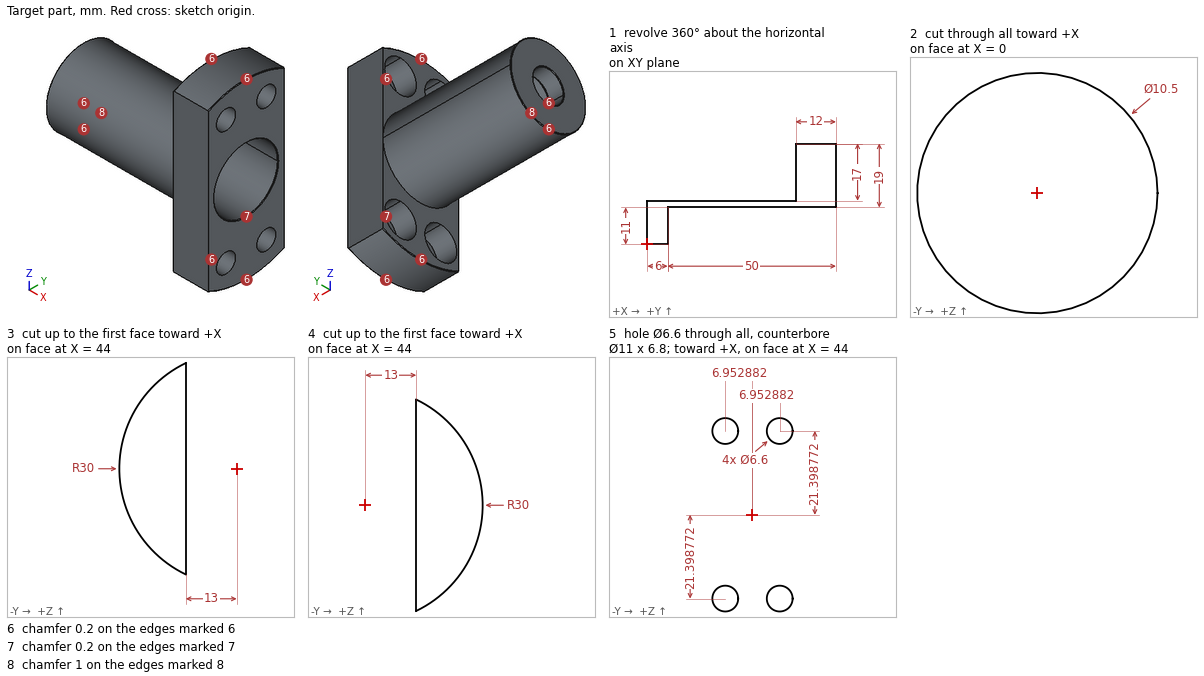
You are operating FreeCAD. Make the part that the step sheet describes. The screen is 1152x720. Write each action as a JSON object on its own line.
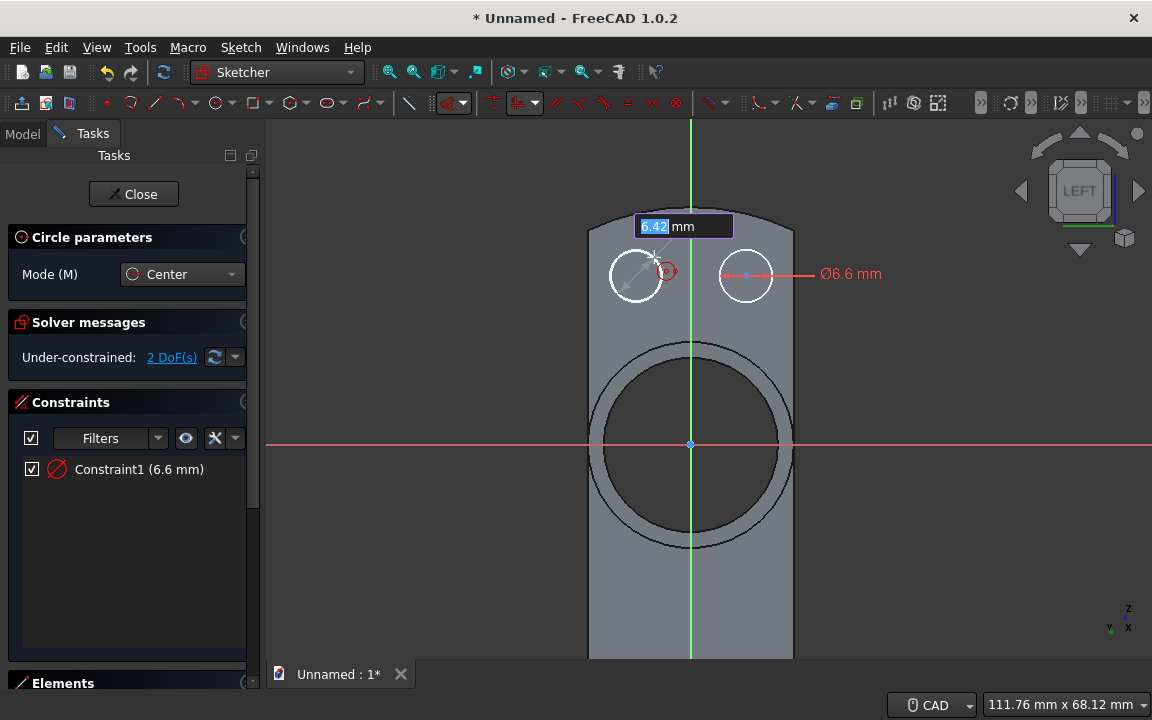
{"action": "type", "text": "6.6"}
{"action": "key", "text": "Return"}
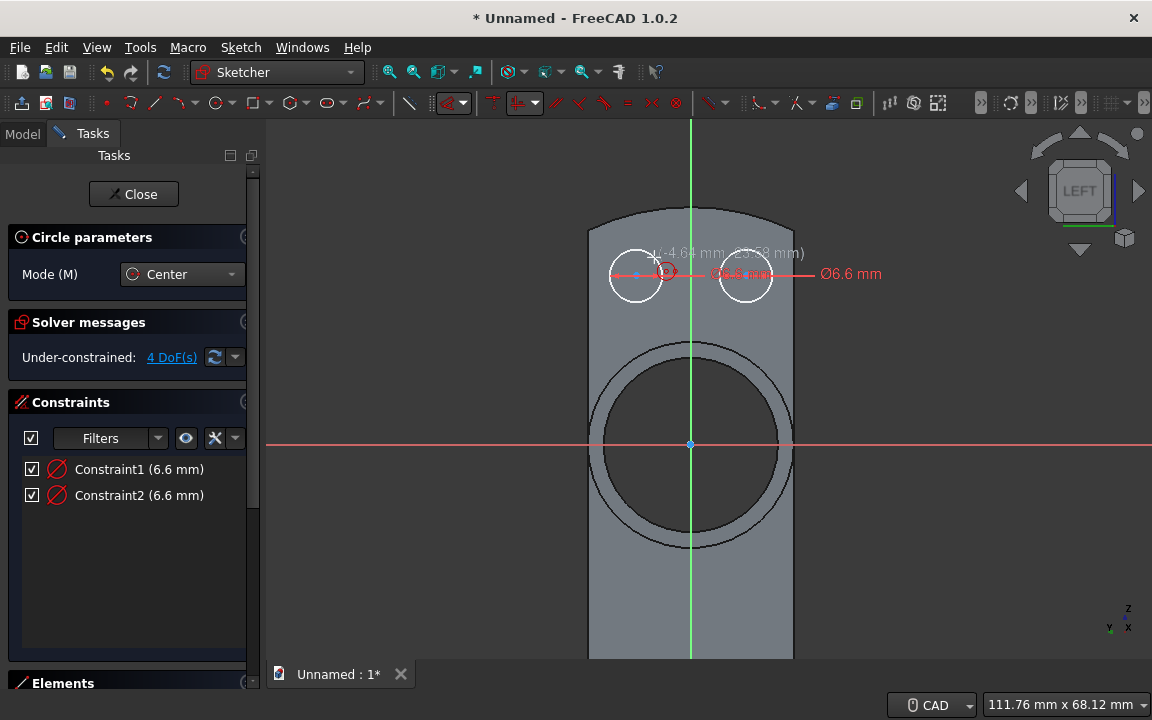
{"action": "left_click", "coordinate": [636, 615]}
{"action": "mouse_move", "coordinate": [654, 596]}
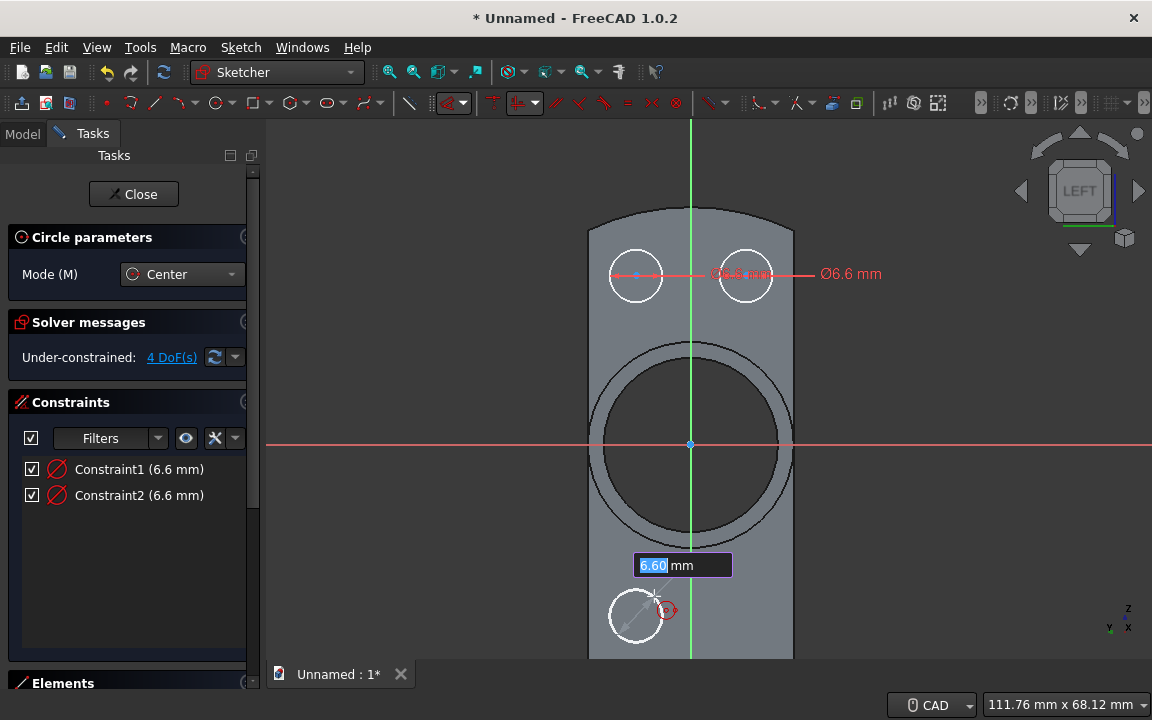
{"action": "type", "text": "6.6"}
{"action": "key", "text": "Return"}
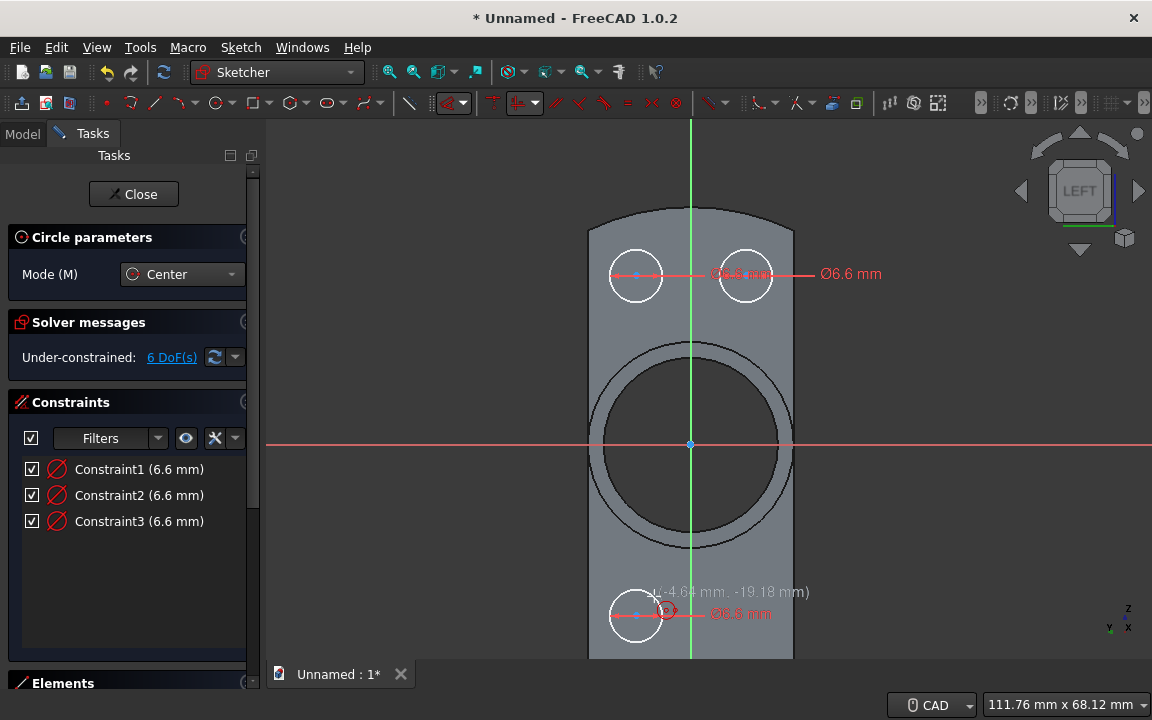
{"action": "left_click", "coordinate": [746, 615]}
{"action": "mouse_move", "coordinate": [764, 596]}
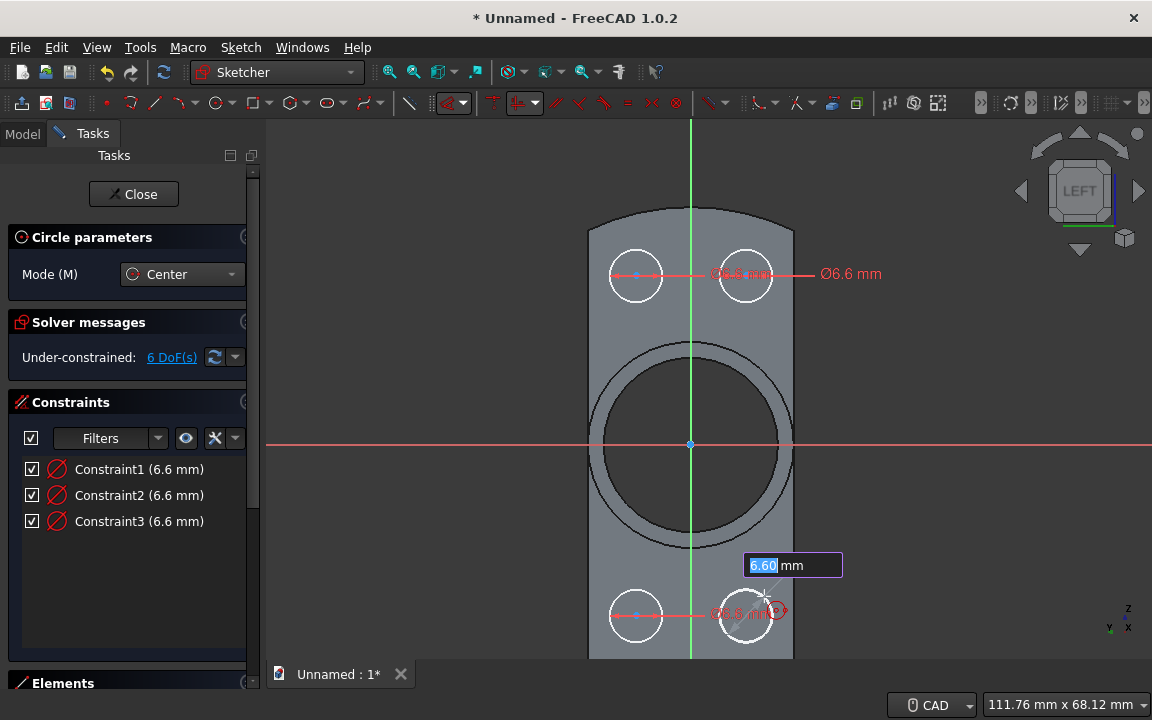
{"action": "type", "text": "6.6"}
{"action": "key", "text": "Return"}
{"action": "key", "text": "Escape"}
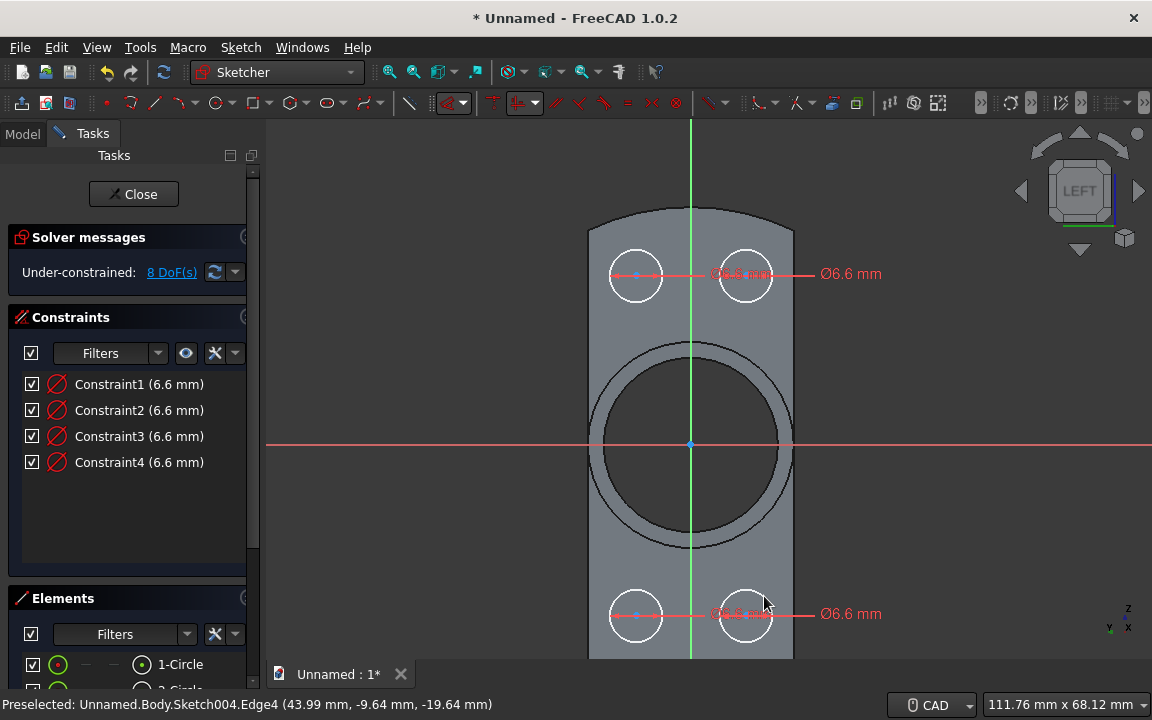
{"action": "left_click", "coordinate": [746, 276]}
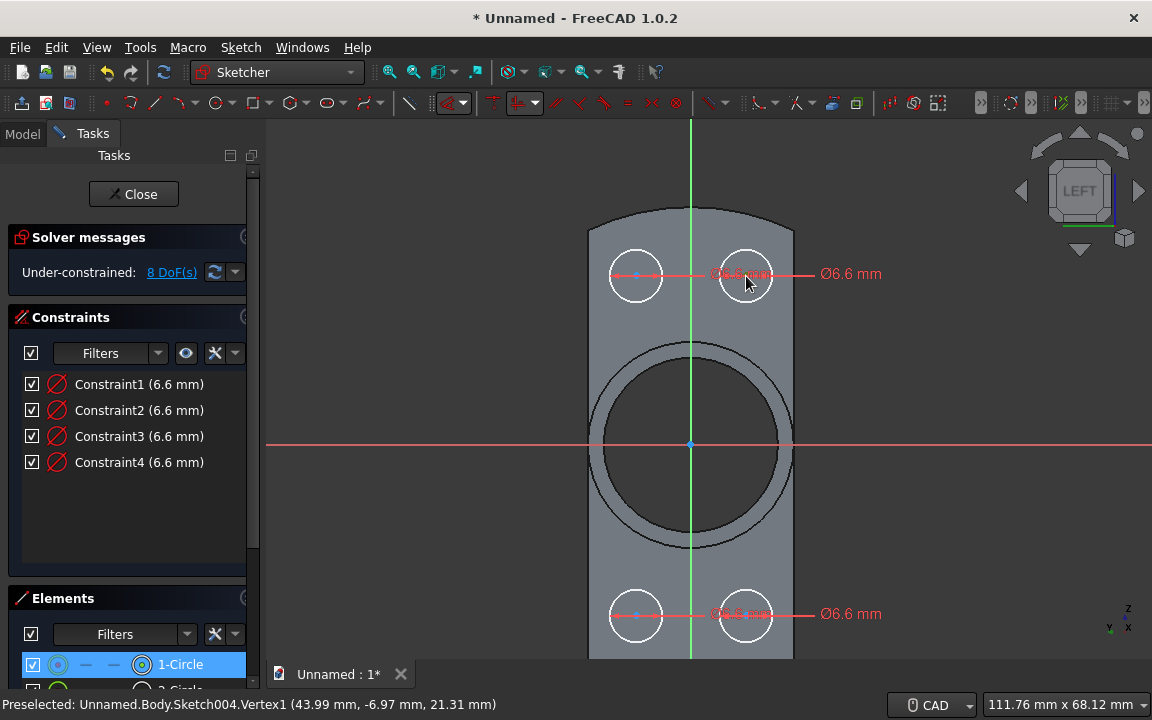
{"action": "left_click", "coordinate": [636, 276]}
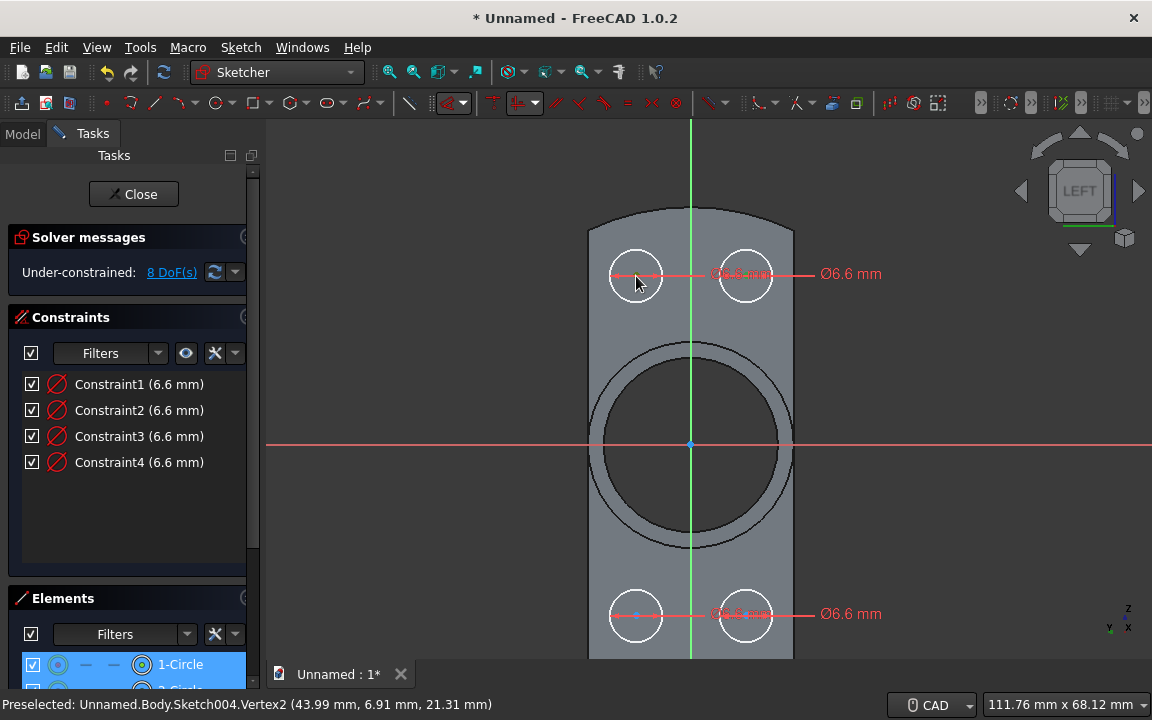
{"action": "key", "text": "h"}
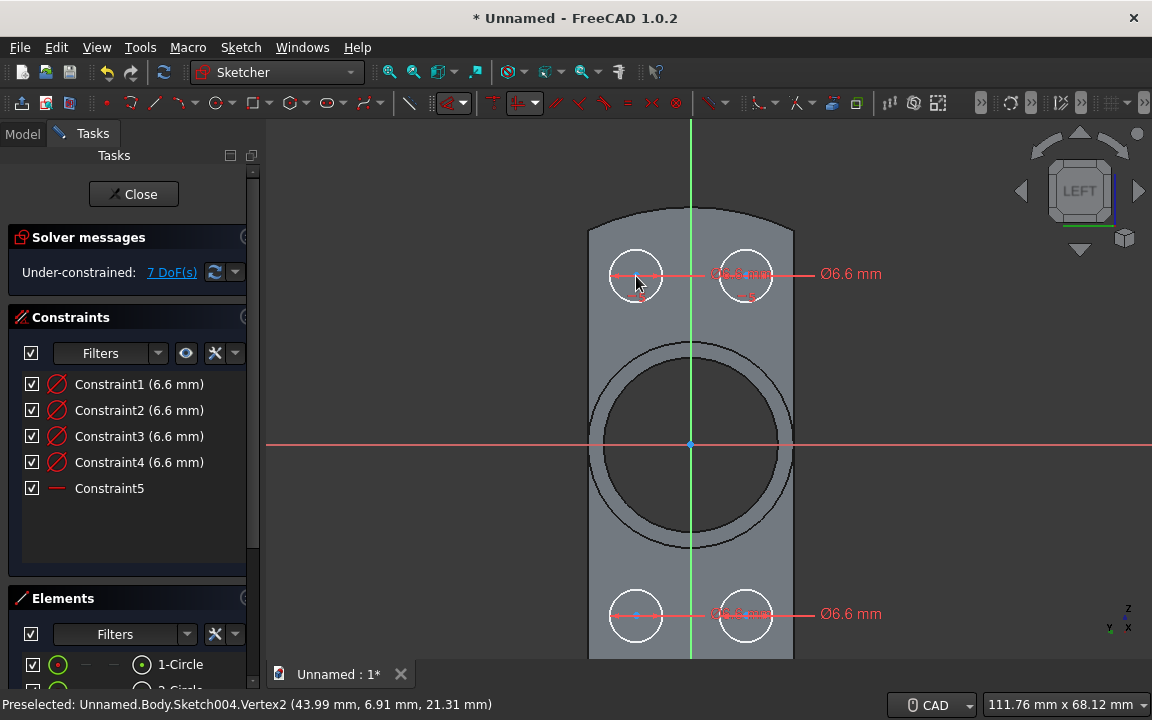
{"action": "left_click", "coordinate": [636, 276]}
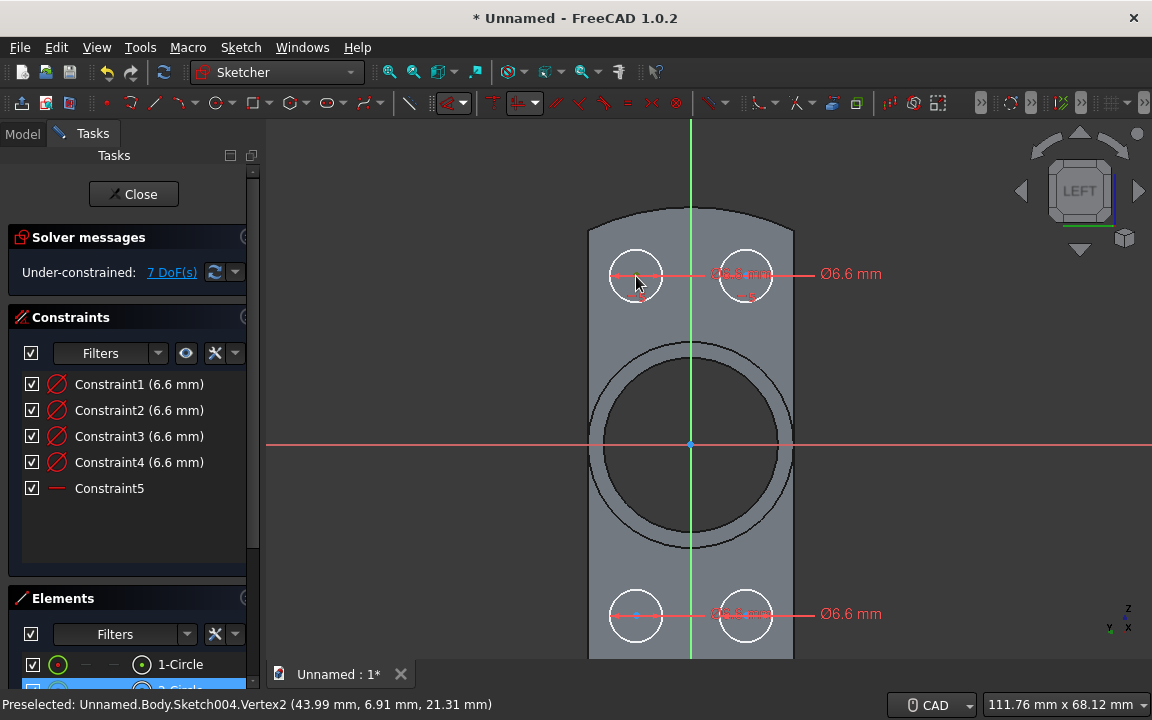
{"action": "left_click", "coordinate": [636, 616]}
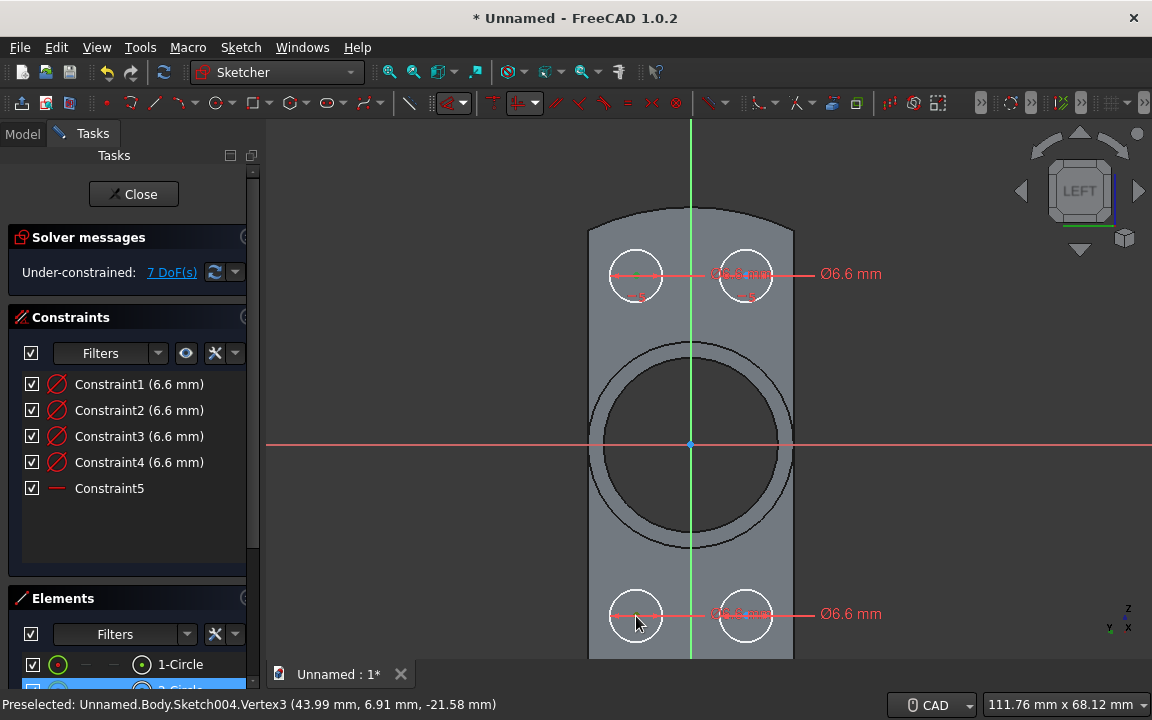
{"action": "key", "text": "v"}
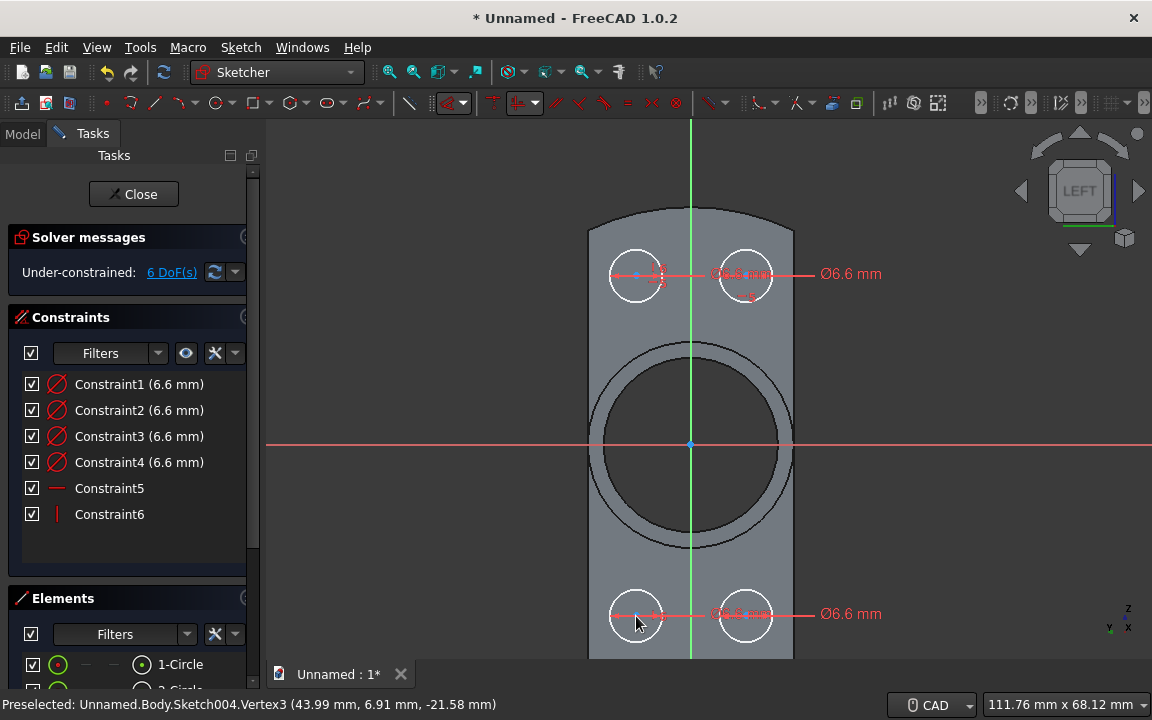
{"action": "left_click", "coordinate": [746, 276]}